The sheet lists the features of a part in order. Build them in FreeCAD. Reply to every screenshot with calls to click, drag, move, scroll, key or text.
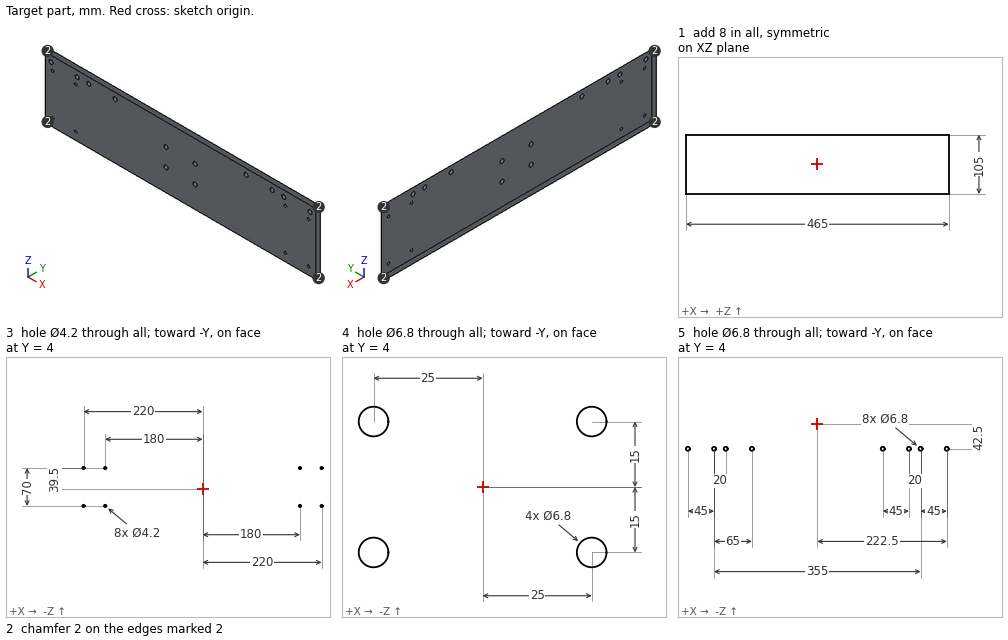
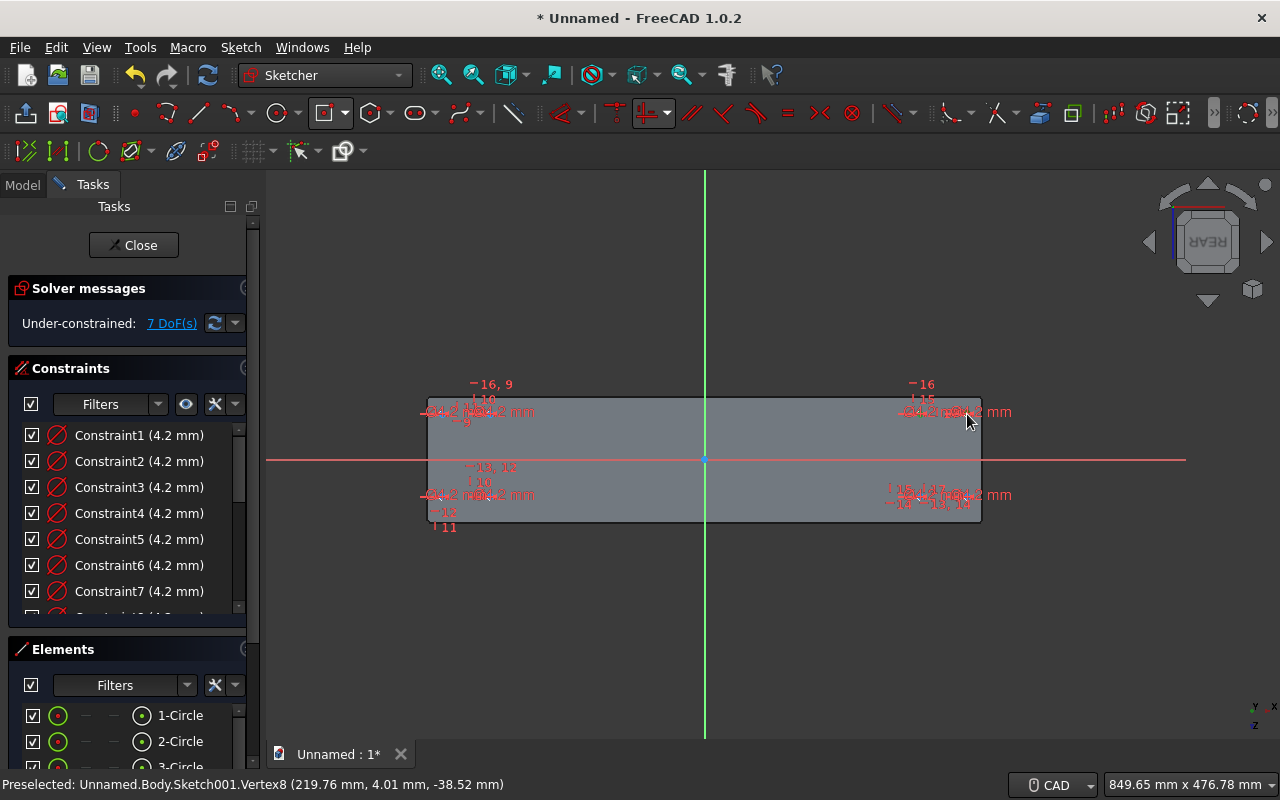
click(670, 114)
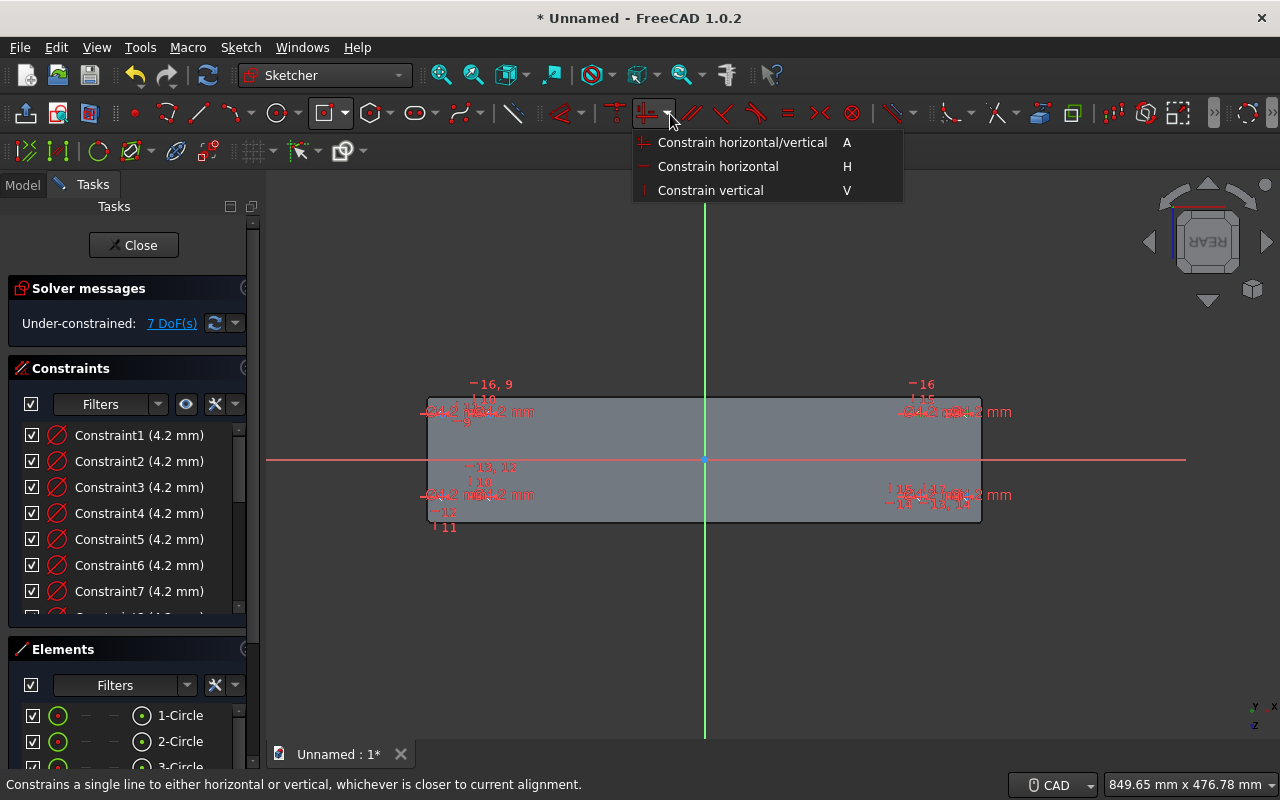
click(768, 166)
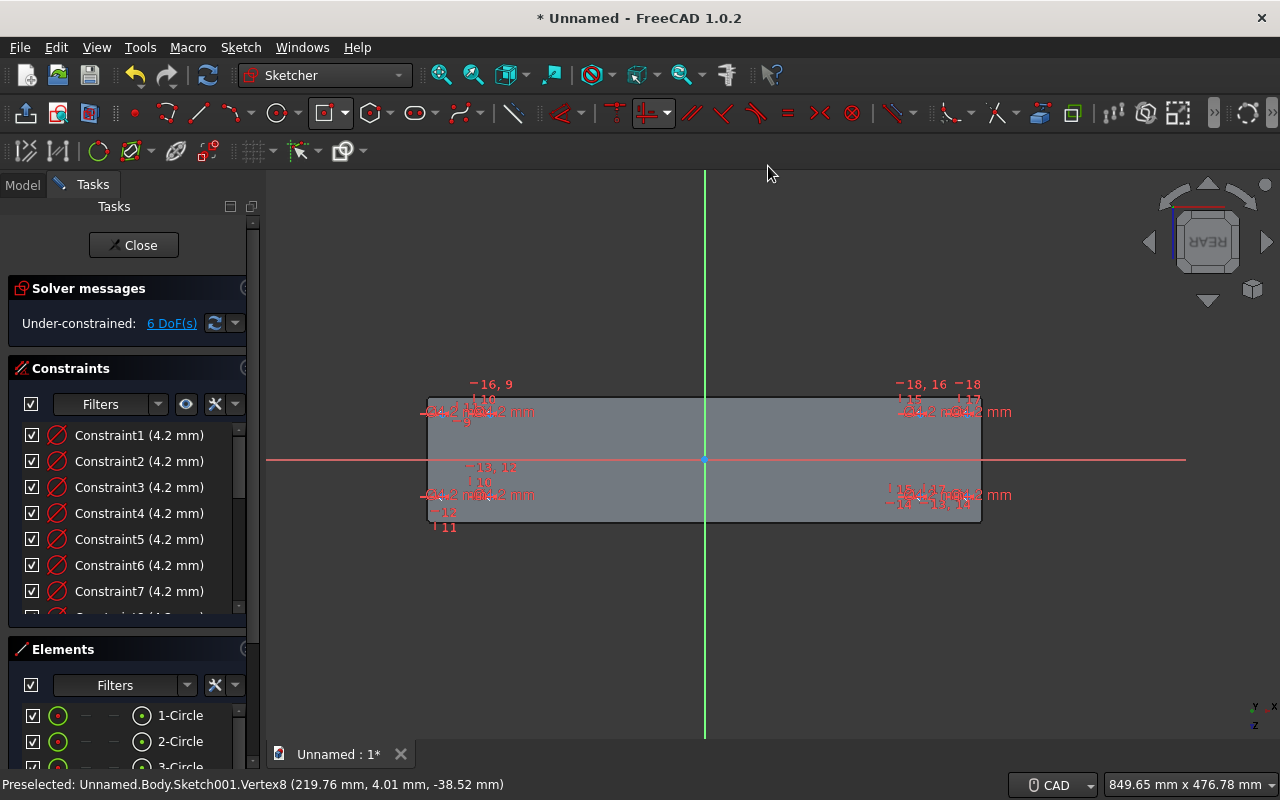
click(442, 414)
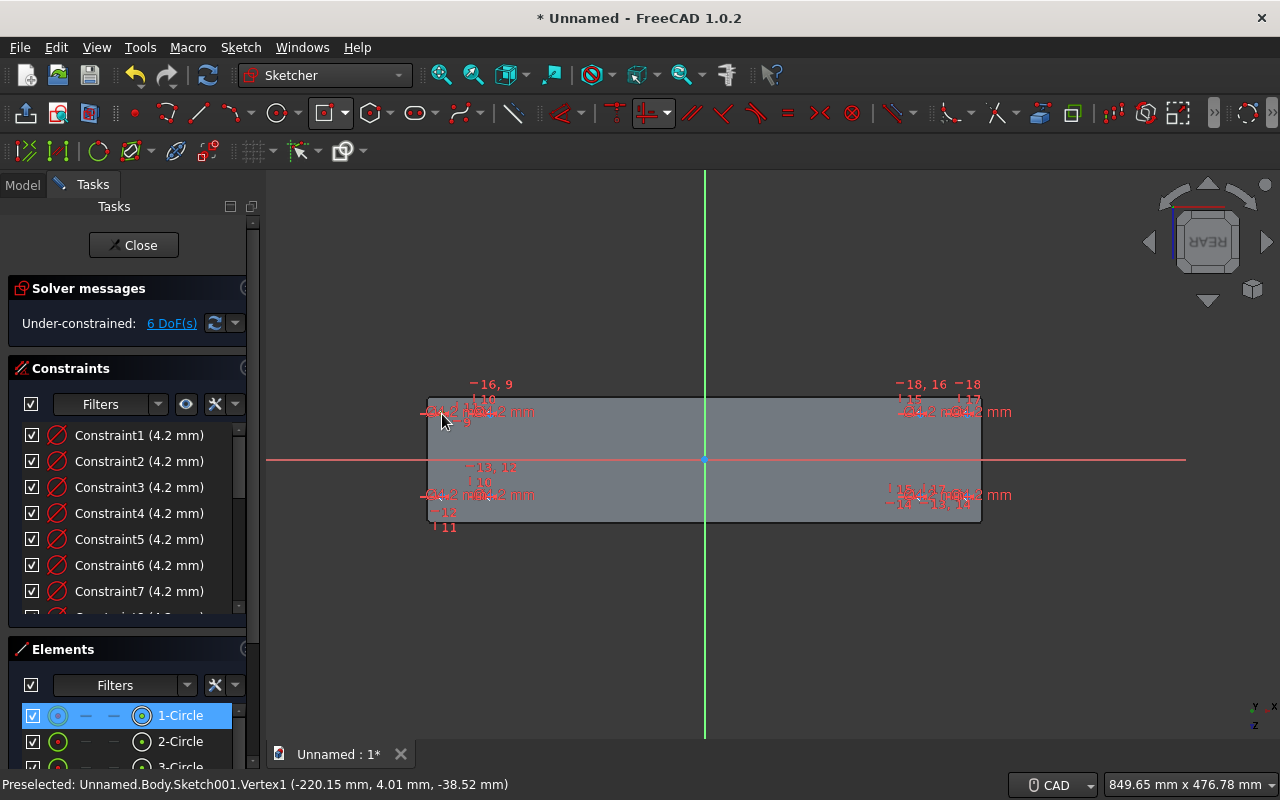
key(l)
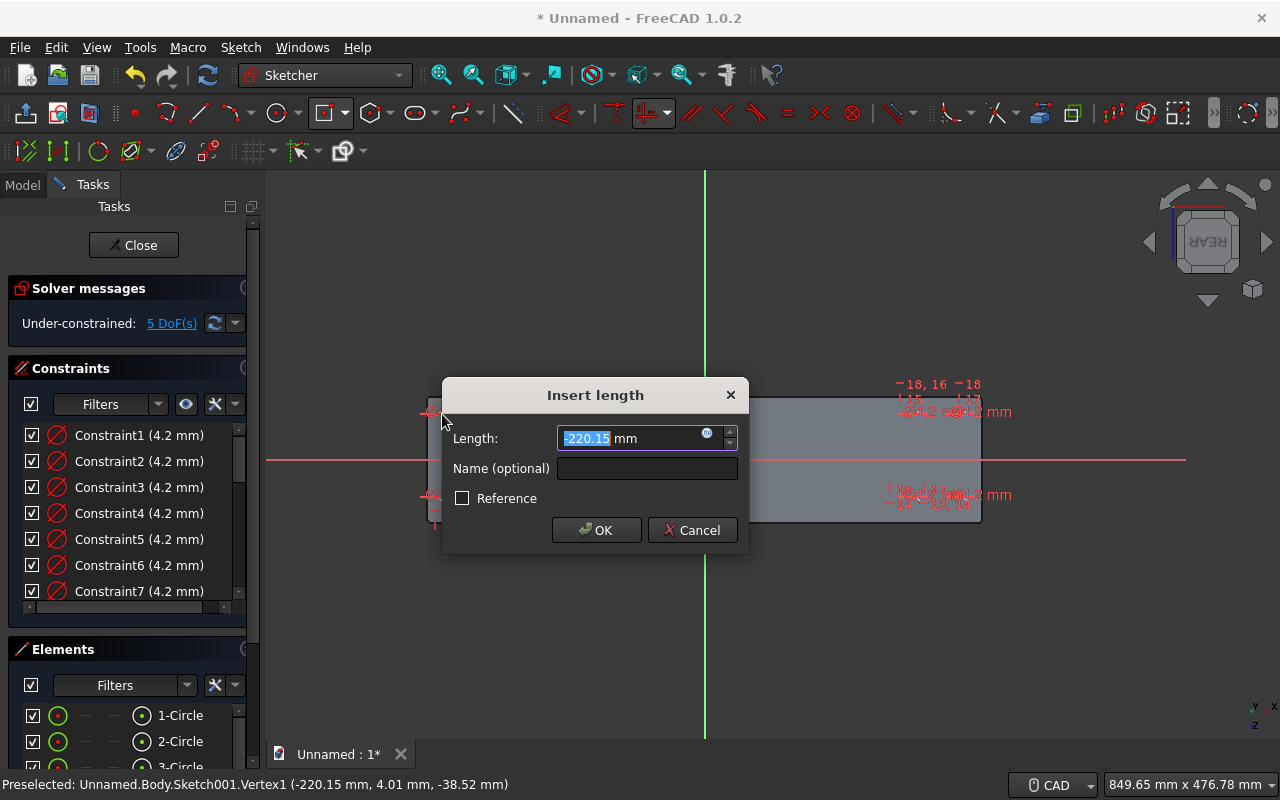
text(-220)
key(Return)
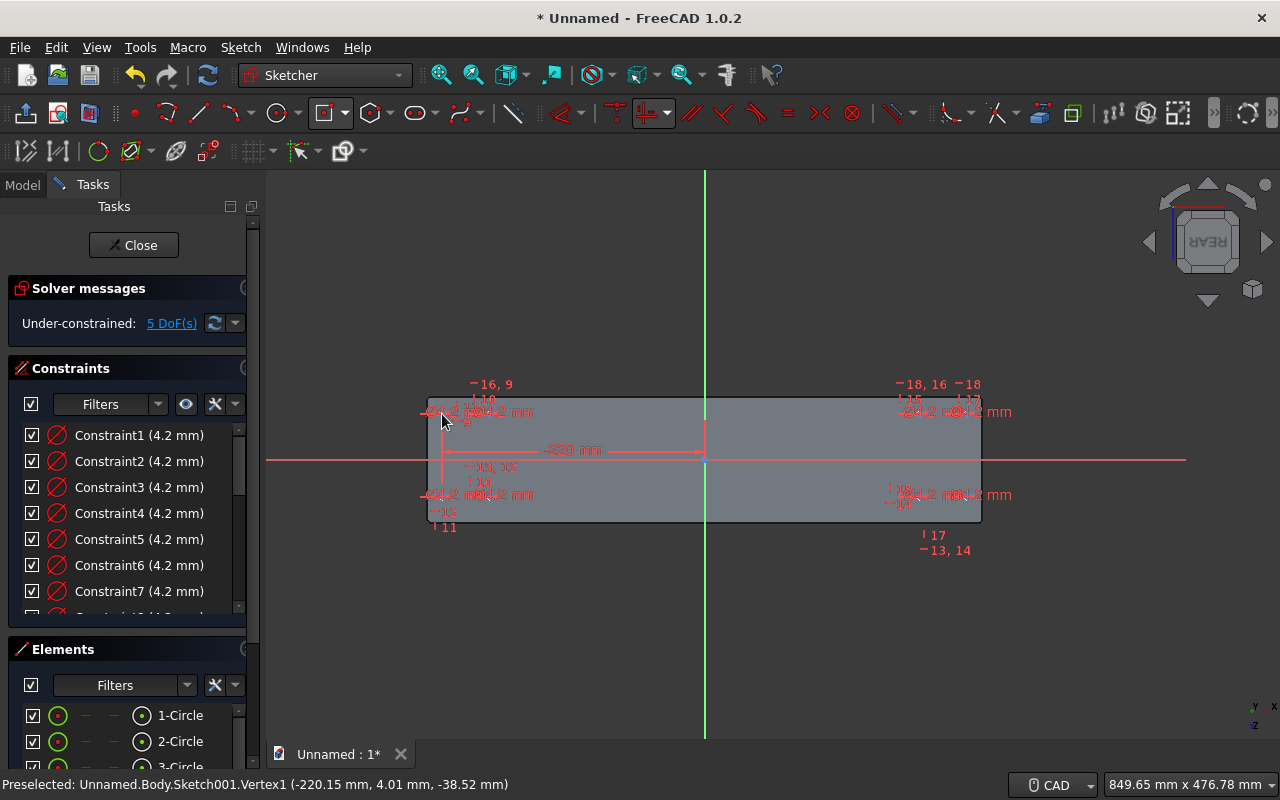
click(490, 414)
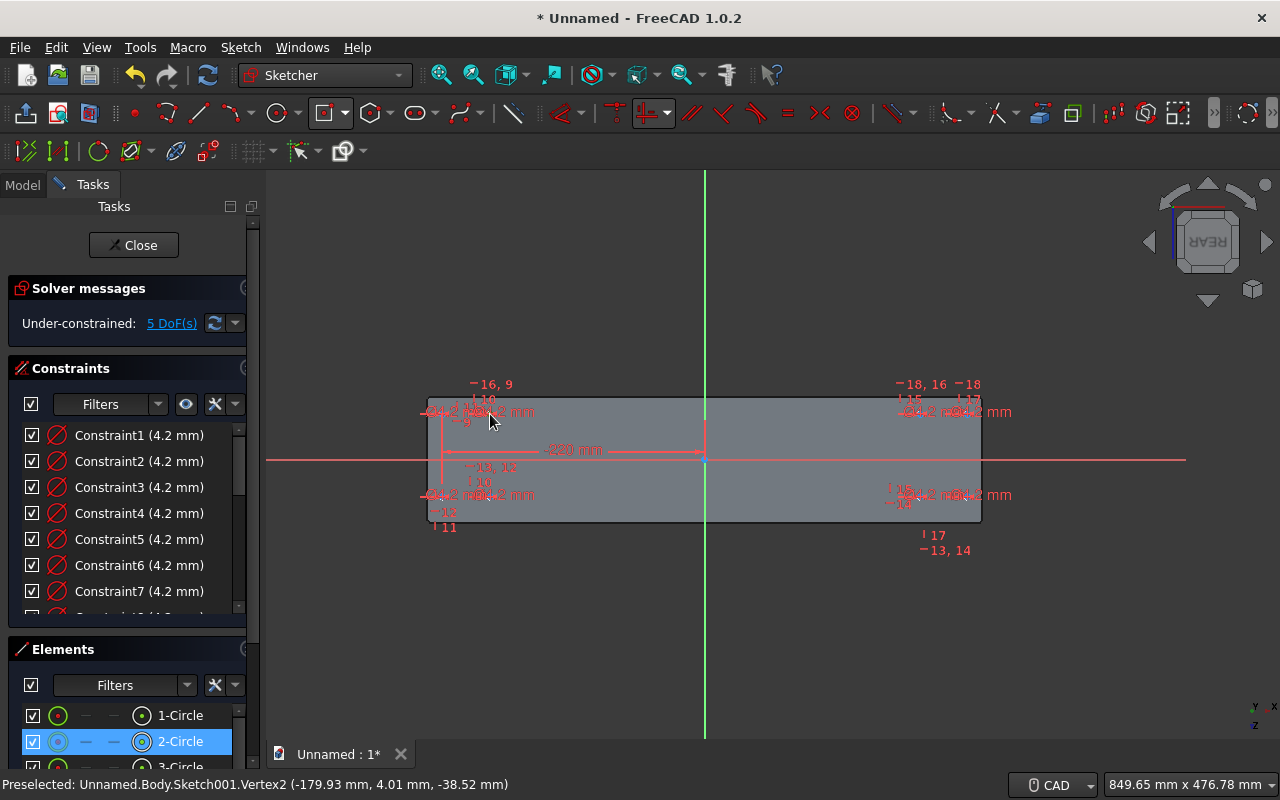
click(584, 114)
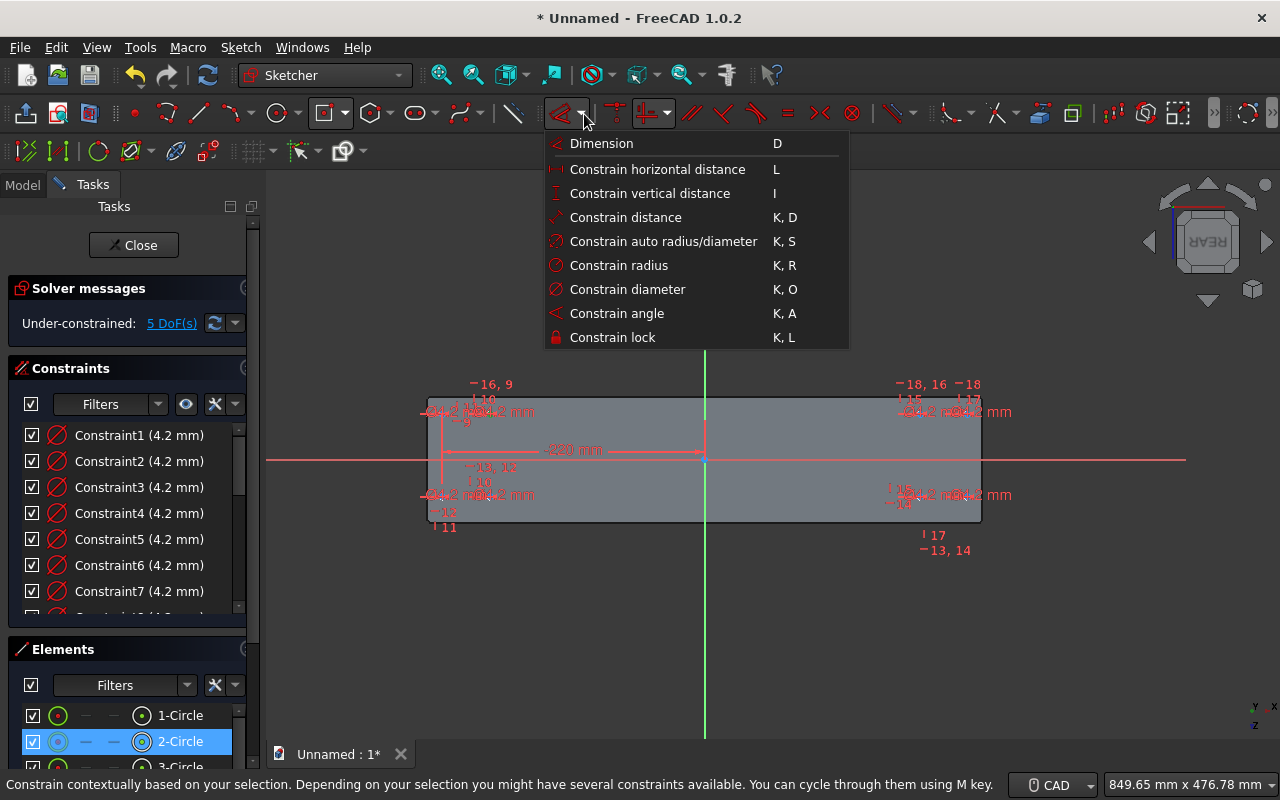
click(697, 169)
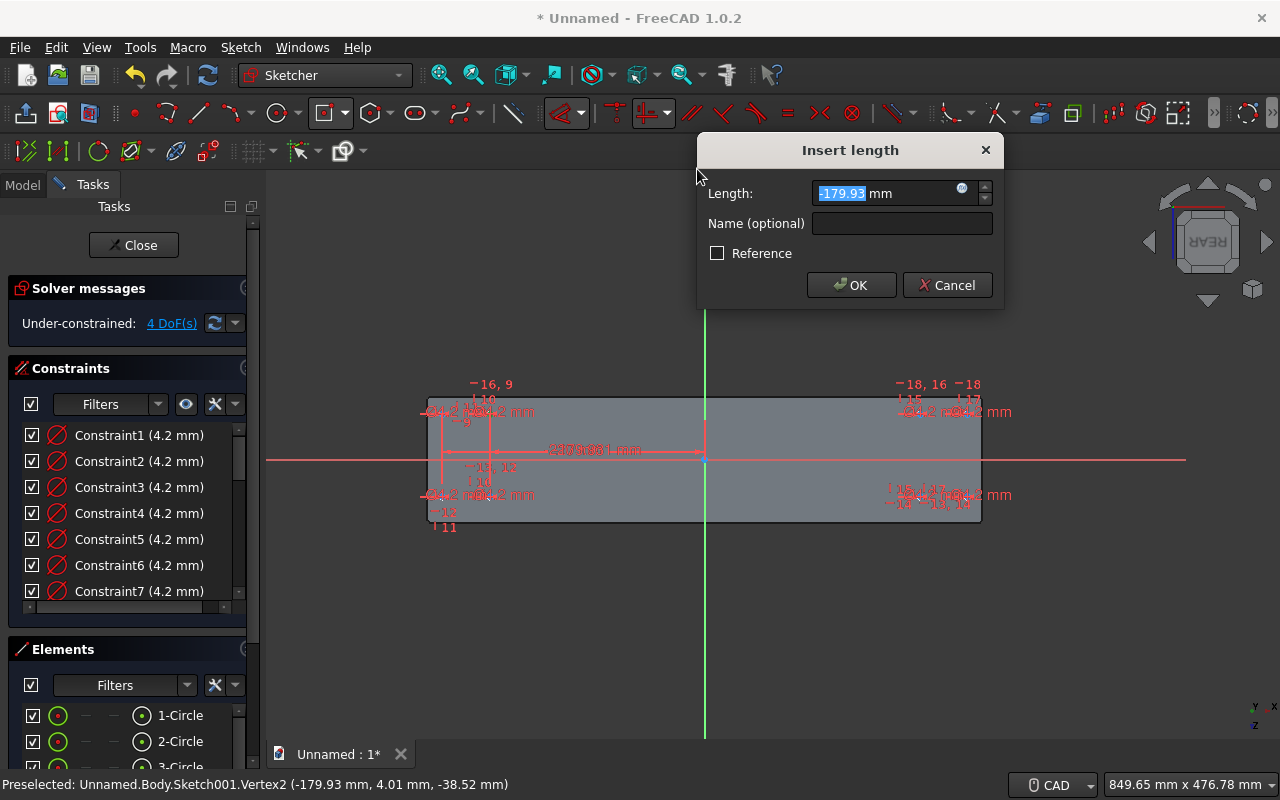
text(-180)
key(Return)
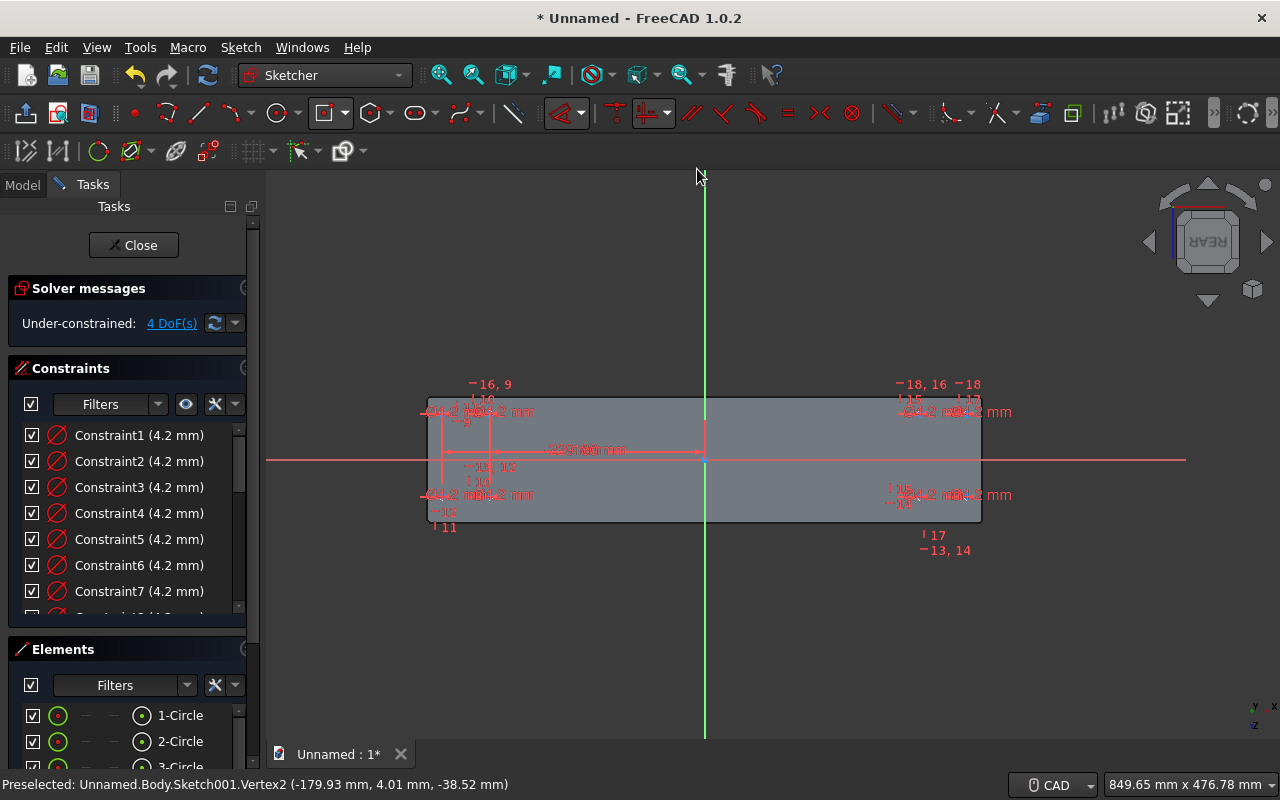
click(967, 497)